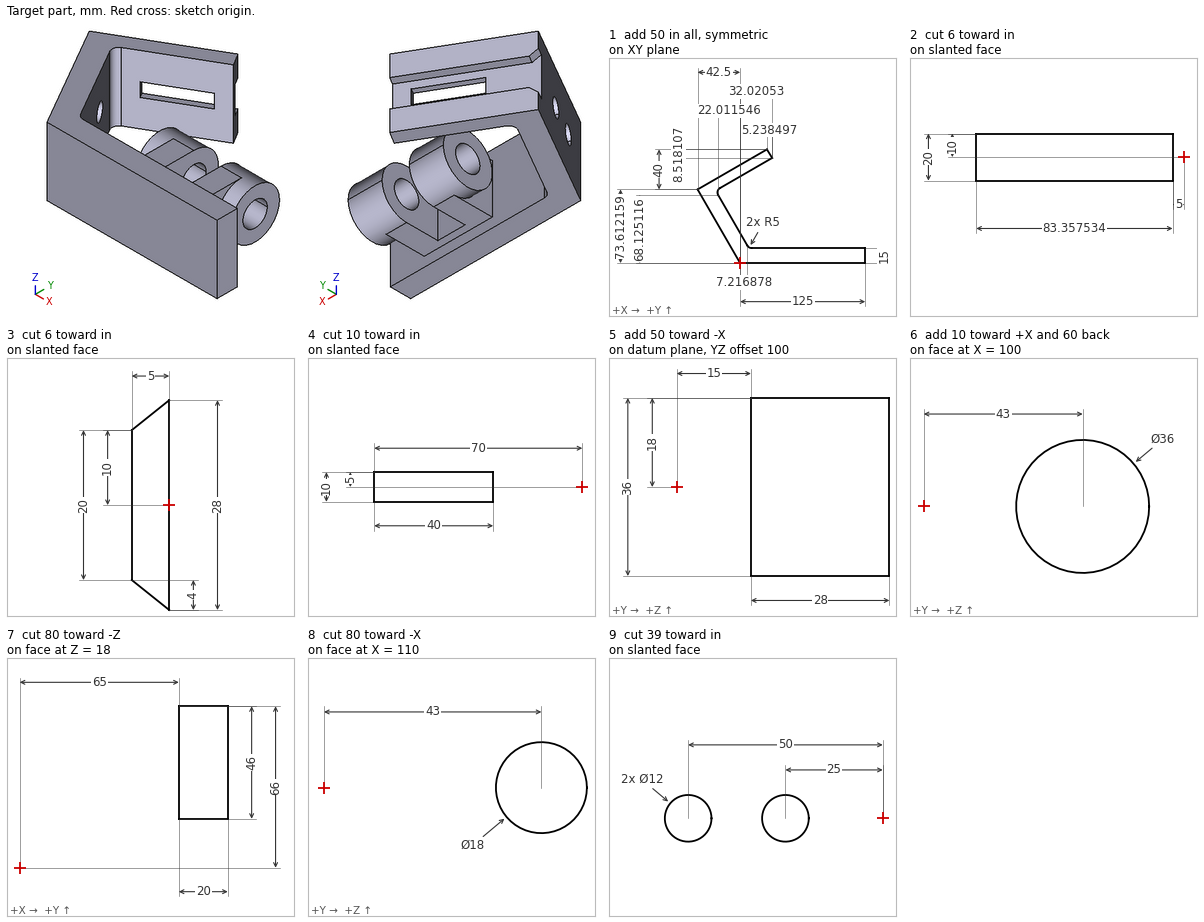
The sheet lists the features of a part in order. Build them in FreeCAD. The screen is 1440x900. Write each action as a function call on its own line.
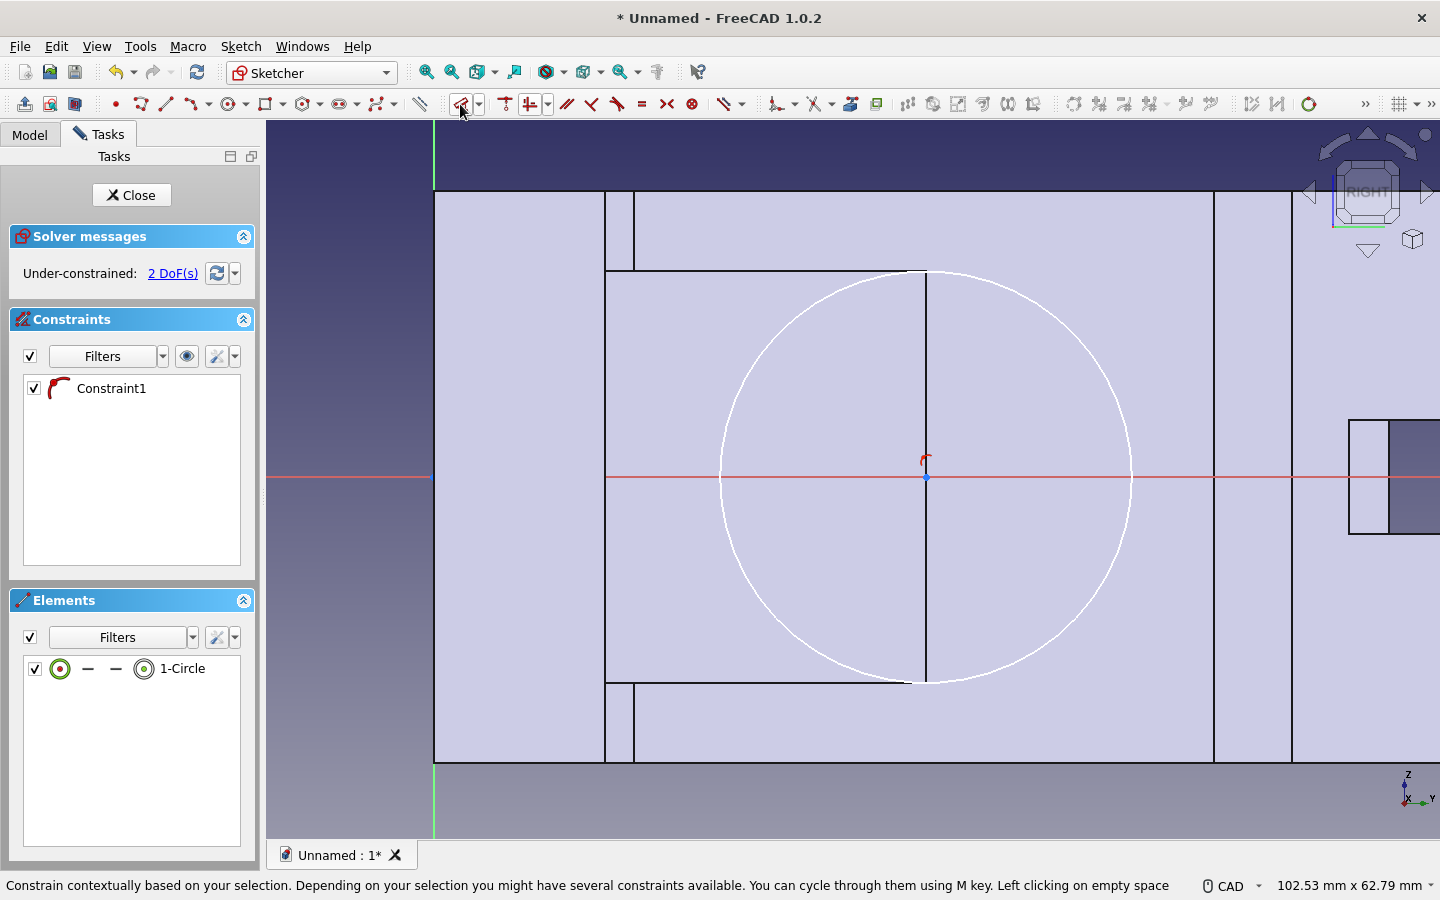
click(1071, 331)
click(1094, 308)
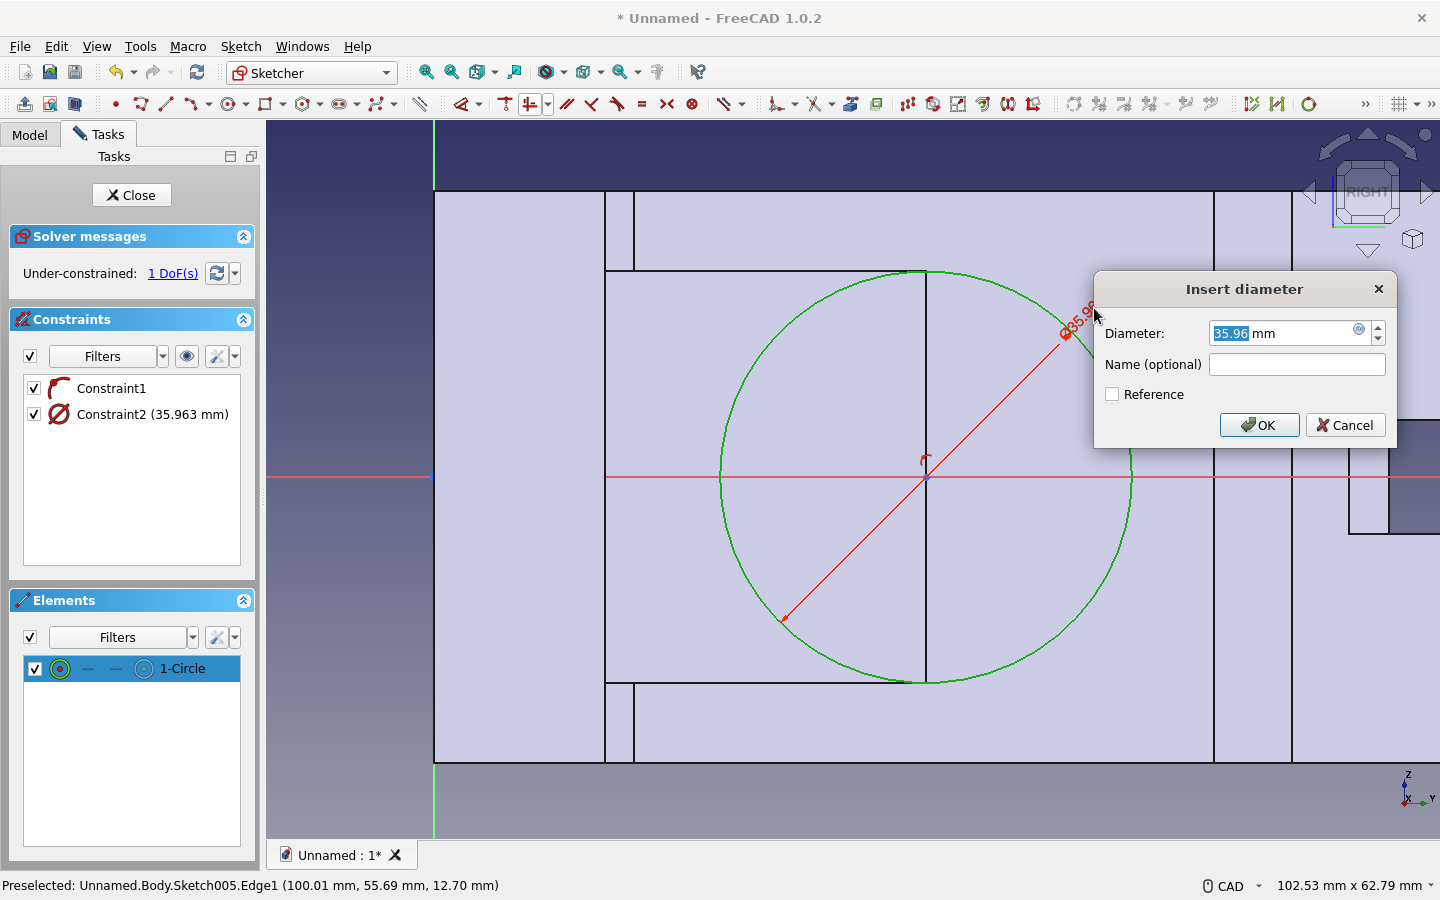
text(36)
key(Return)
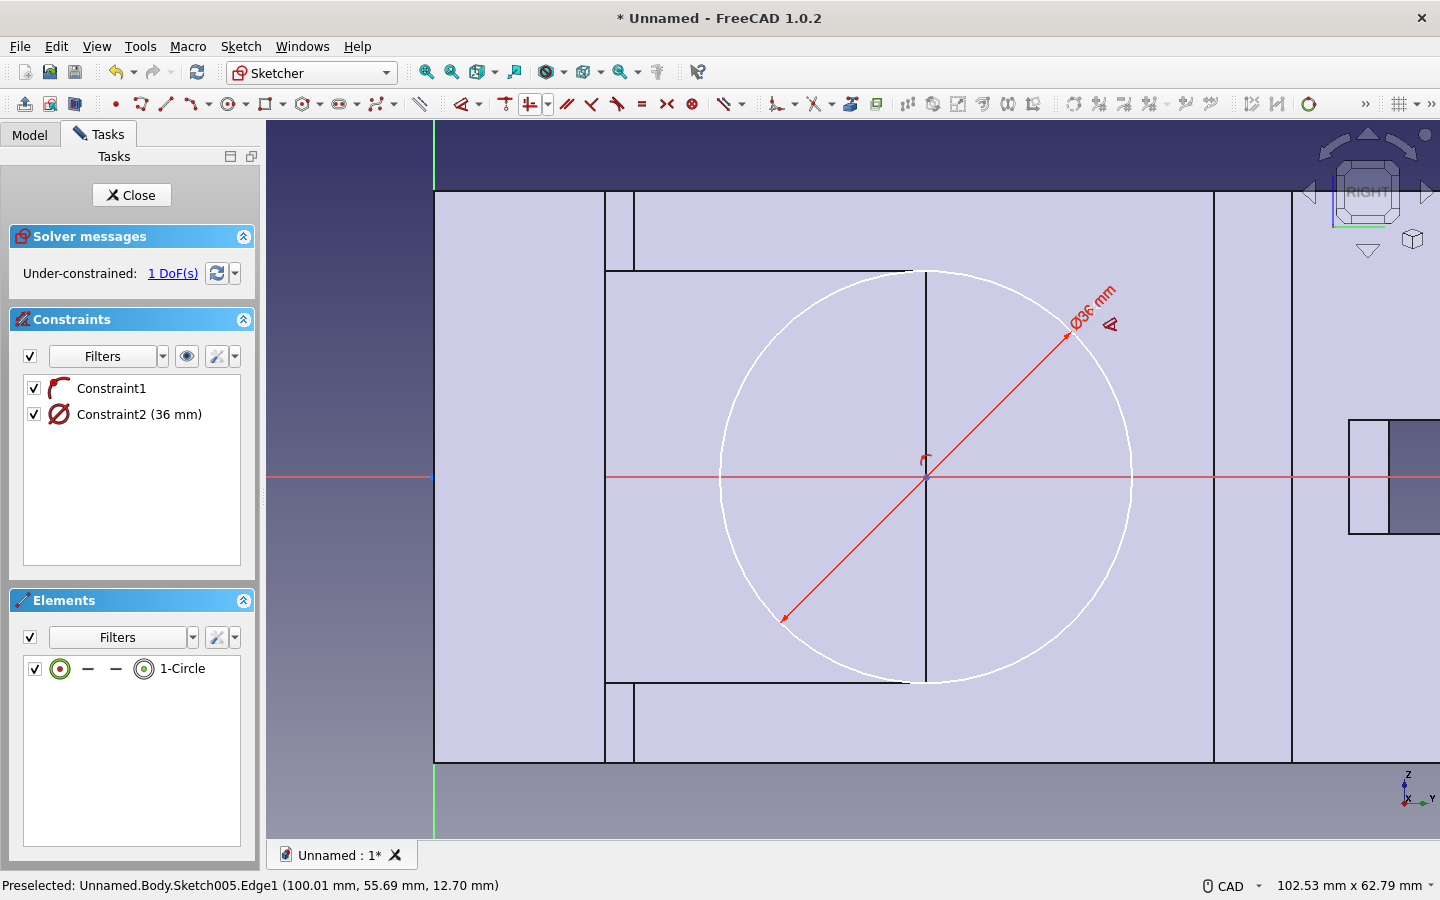
click(926, 477)
click(680, 511)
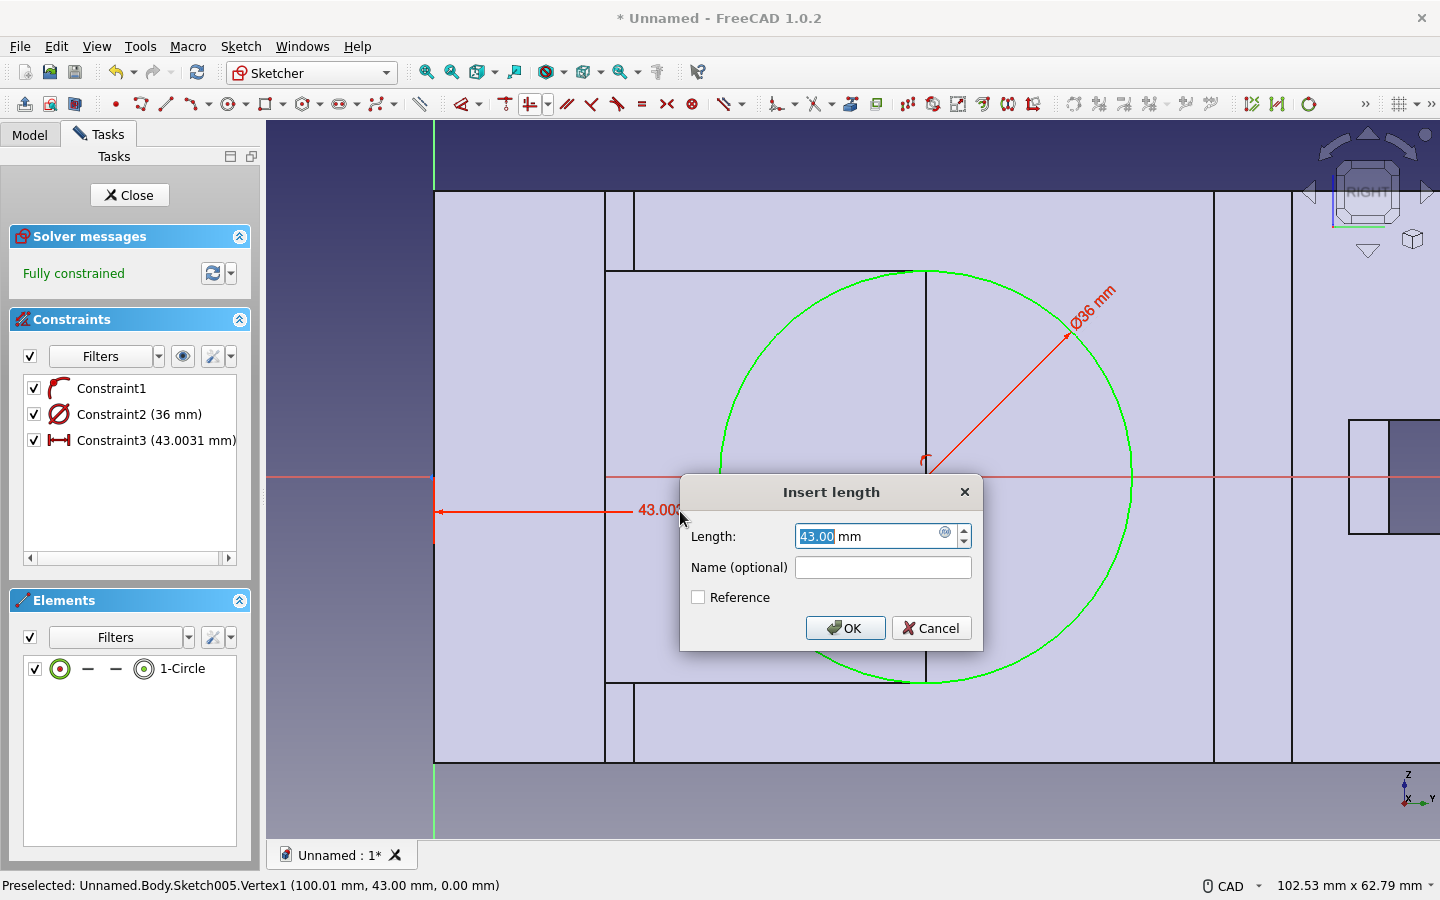
text(43)
key(Return)
key(Escape)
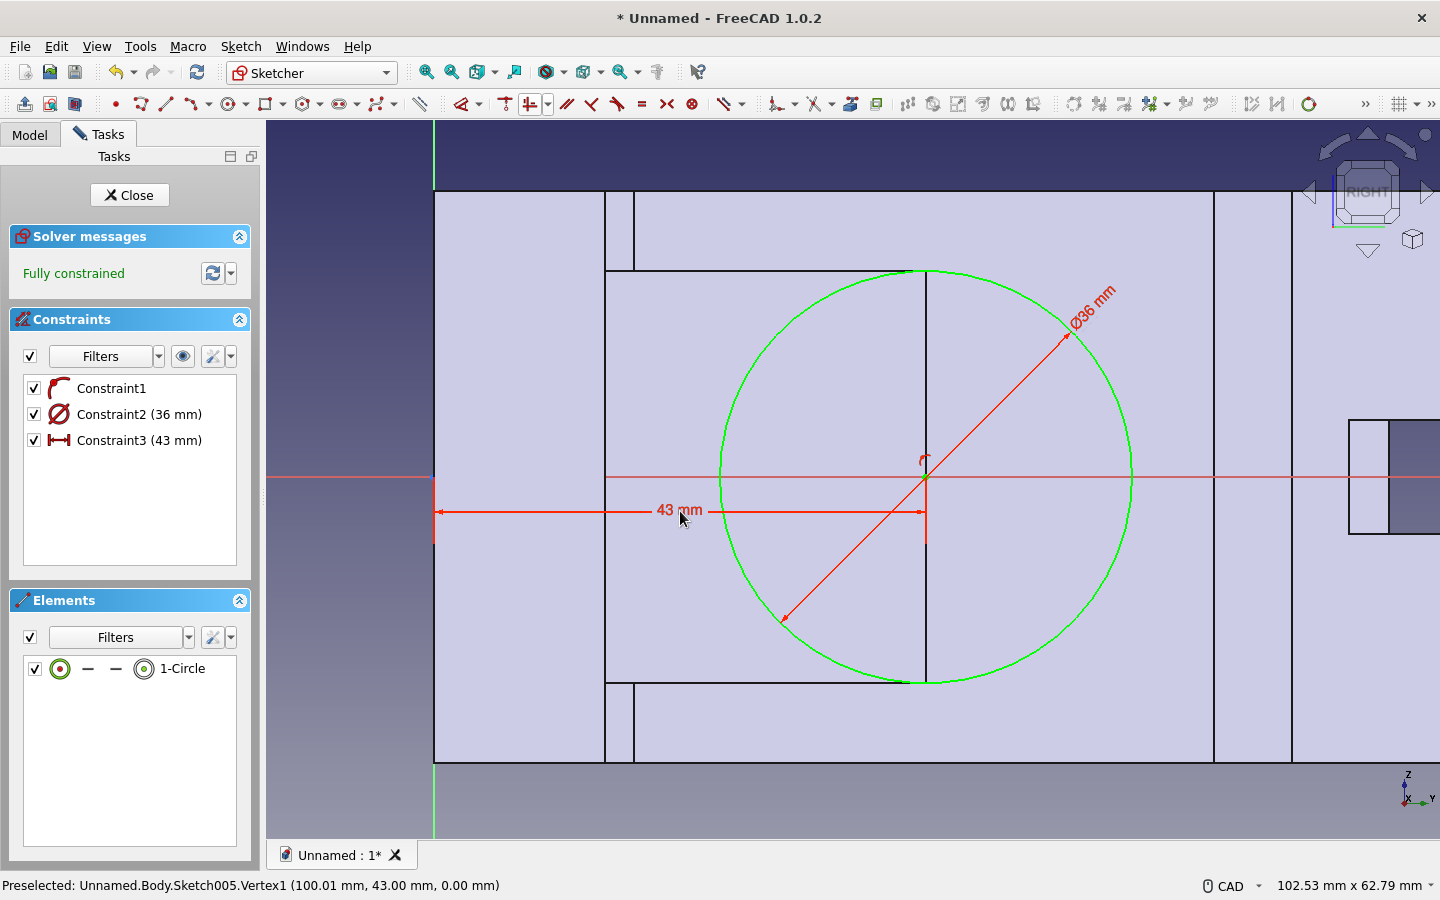
click(130, 195)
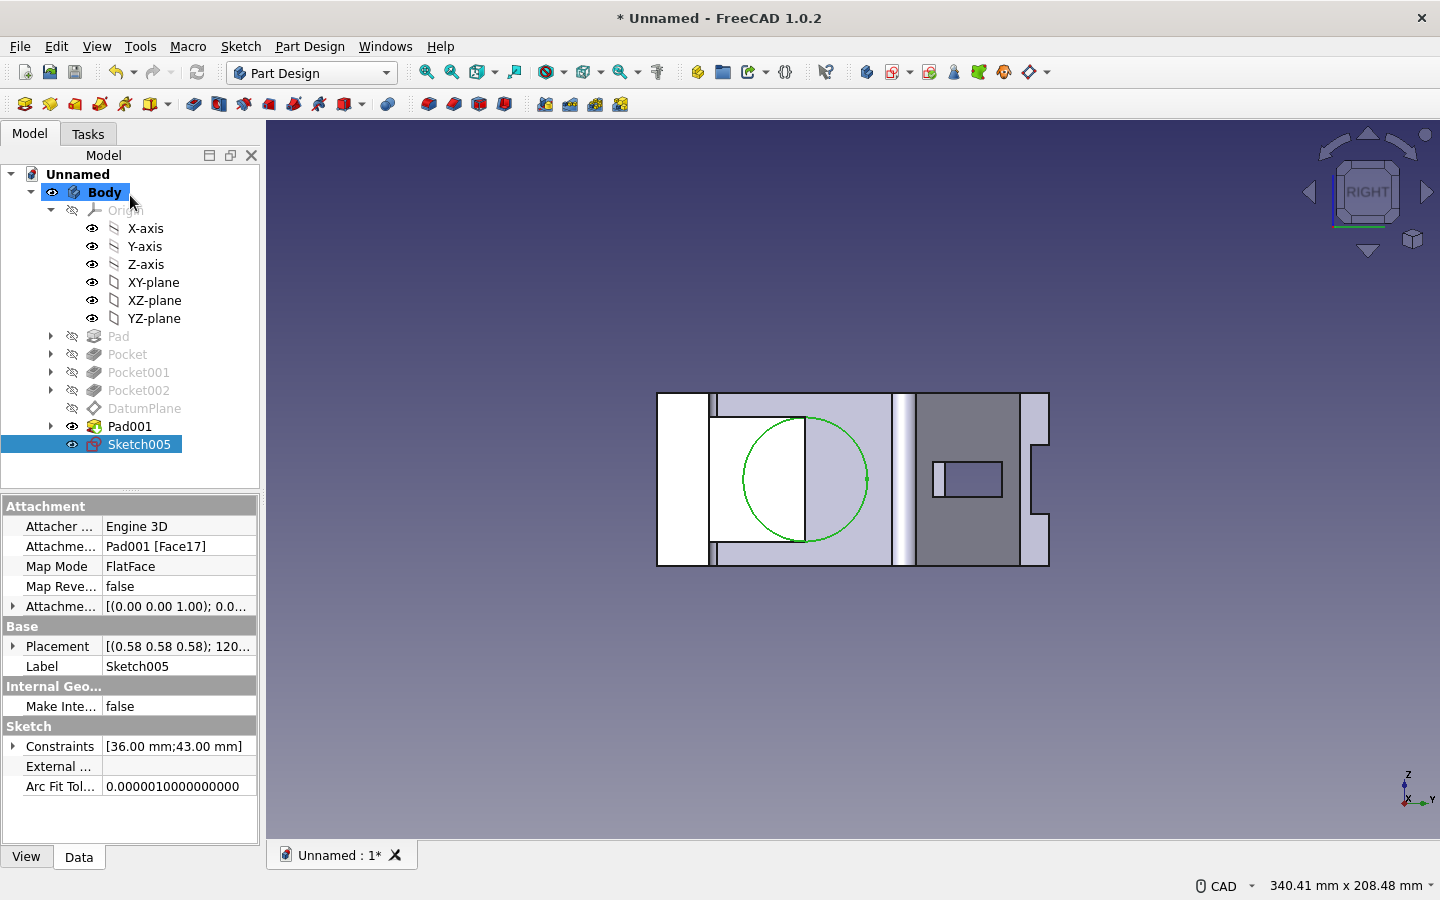
click(25, 104)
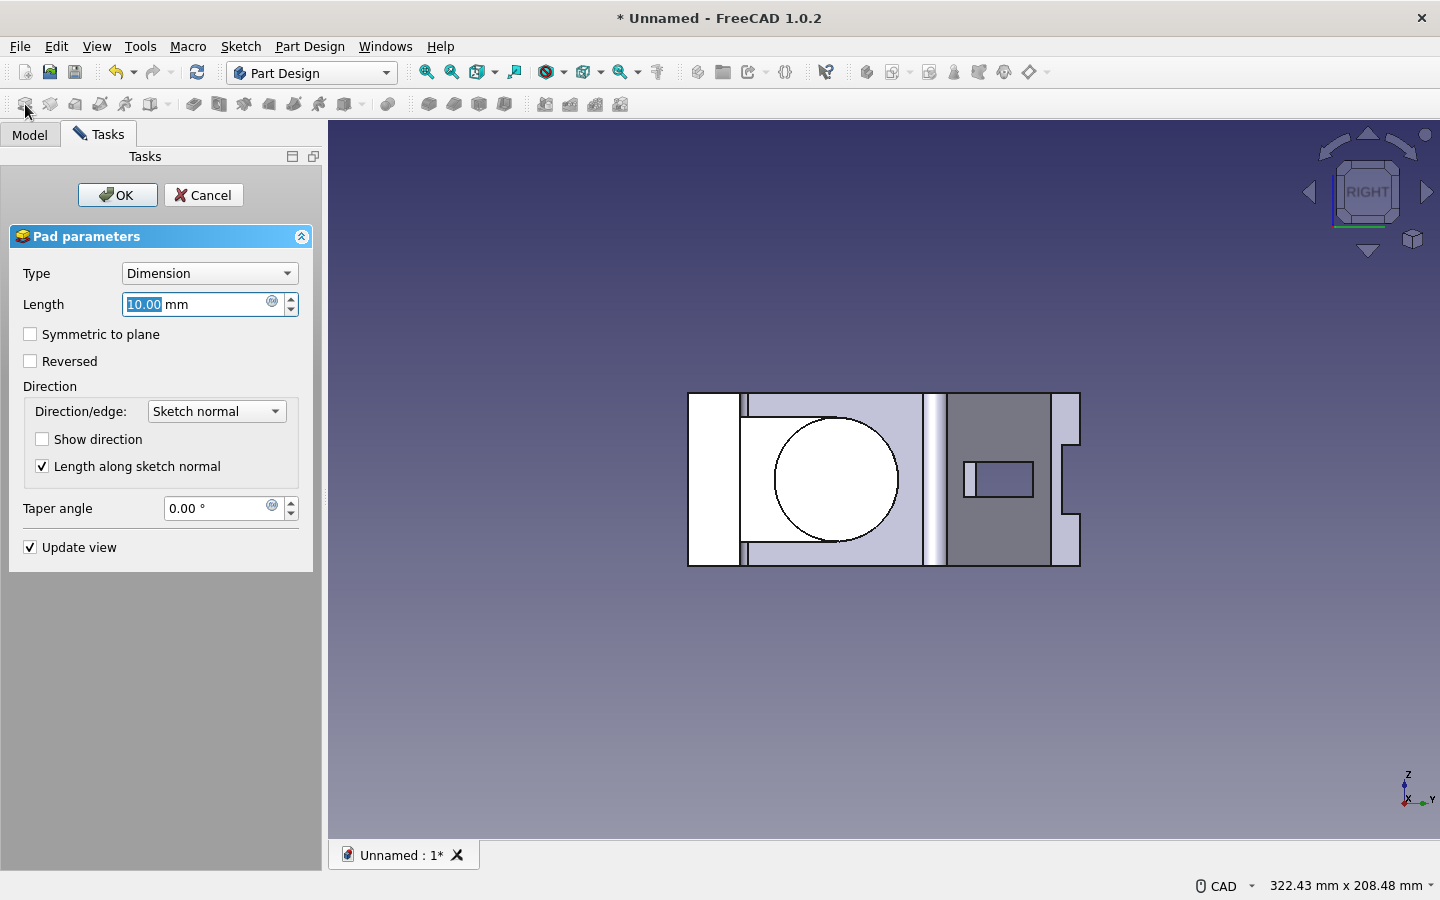
click(210, 274)